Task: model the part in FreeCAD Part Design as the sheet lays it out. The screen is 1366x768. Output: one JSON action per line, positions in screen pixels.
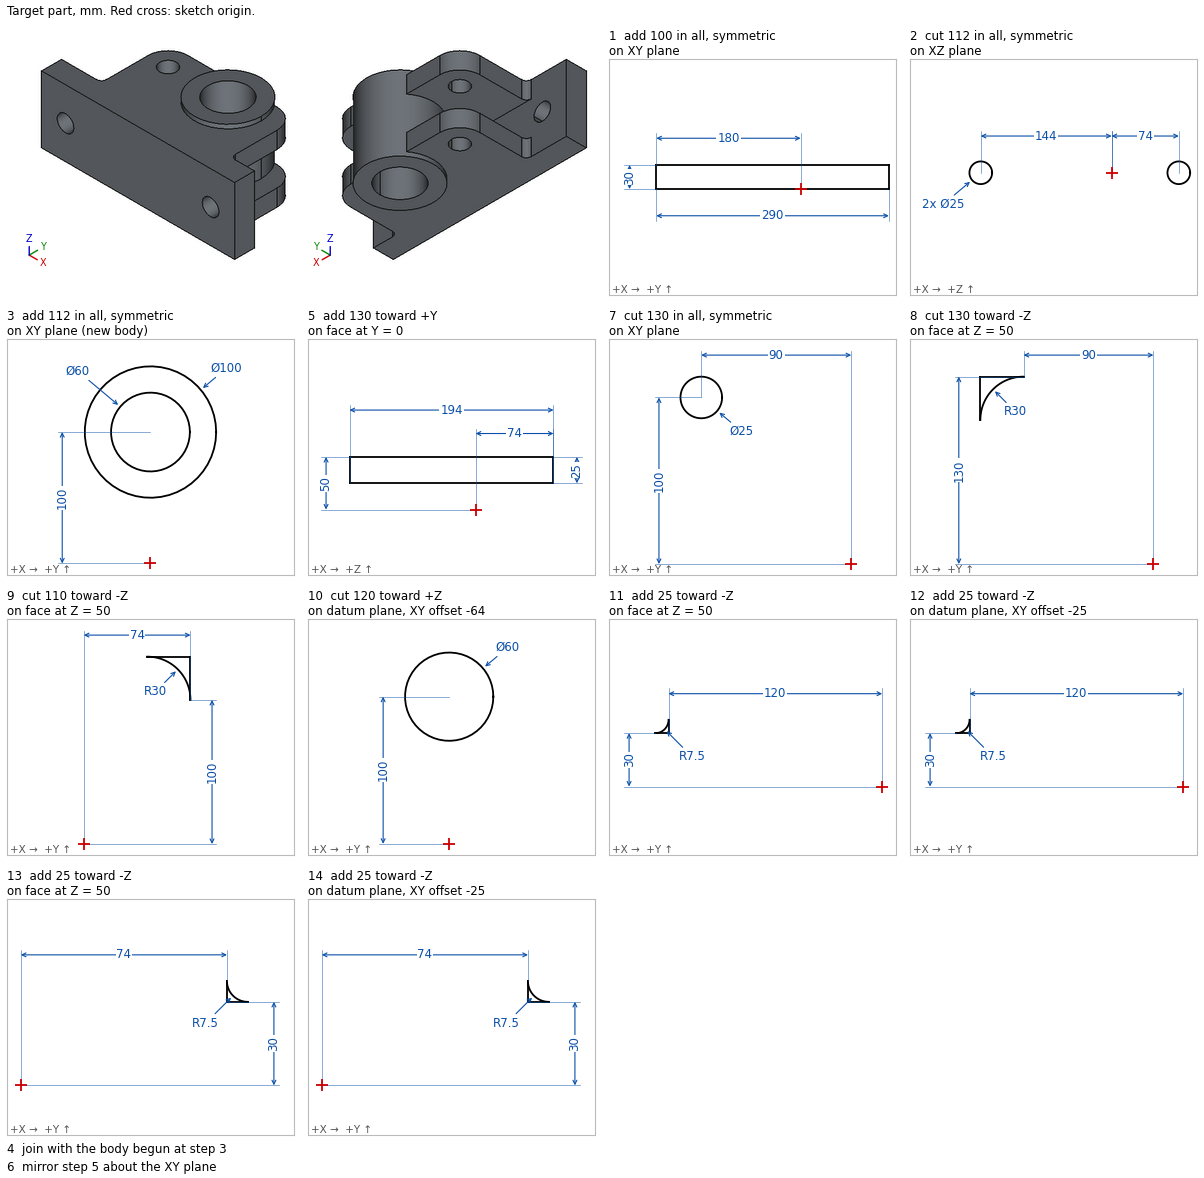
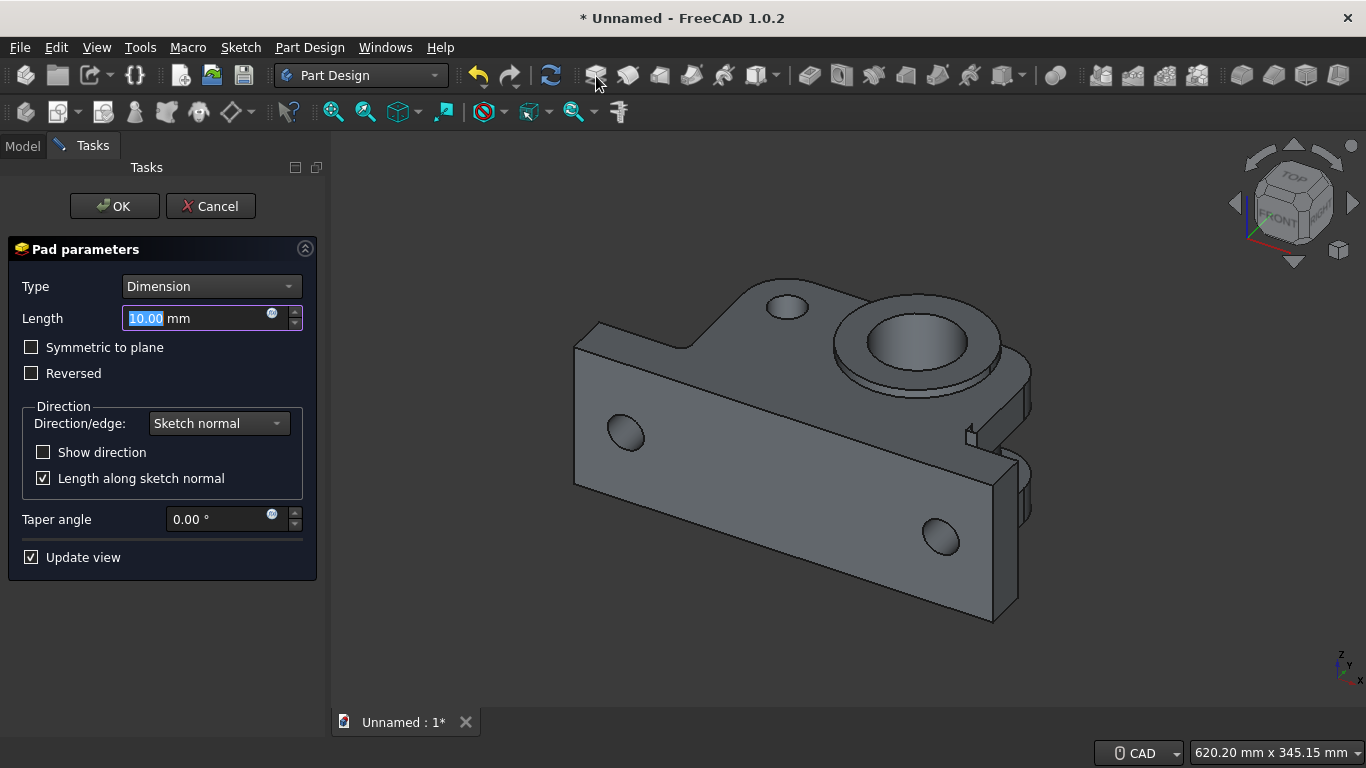
{"action": "type", "text": "25"}
{"action": "key", "text": "Tab"}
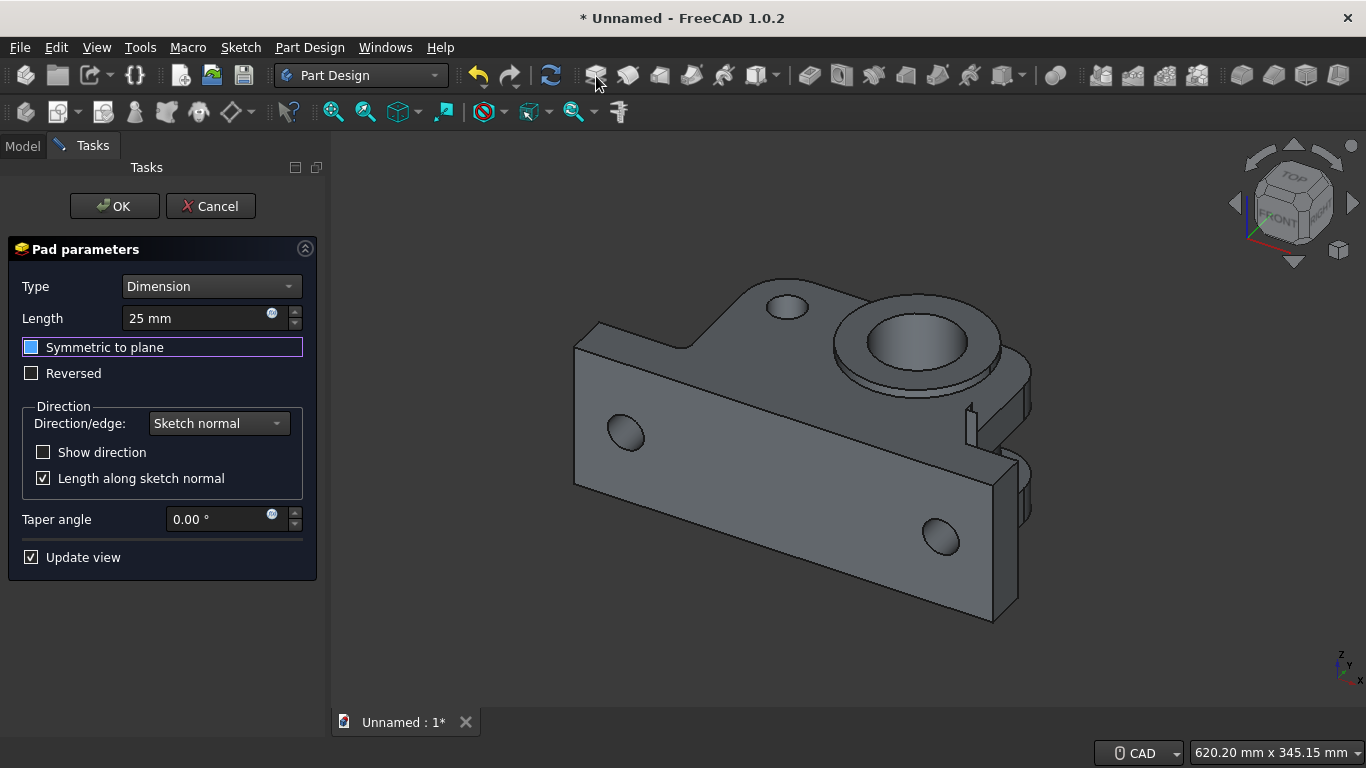
{"action": "left_click", "coordinate": [30, 373]}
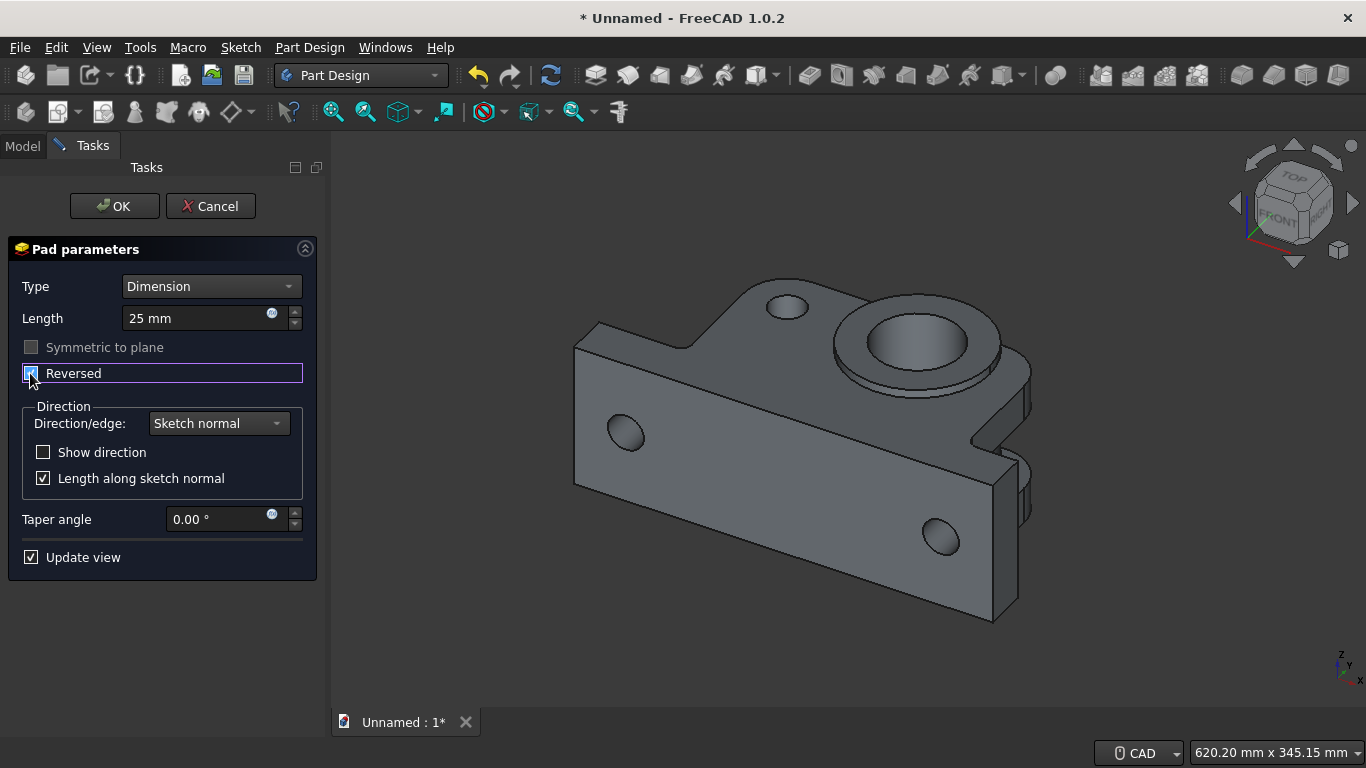
{"action": "left_click", "coordinate": [115, 206]}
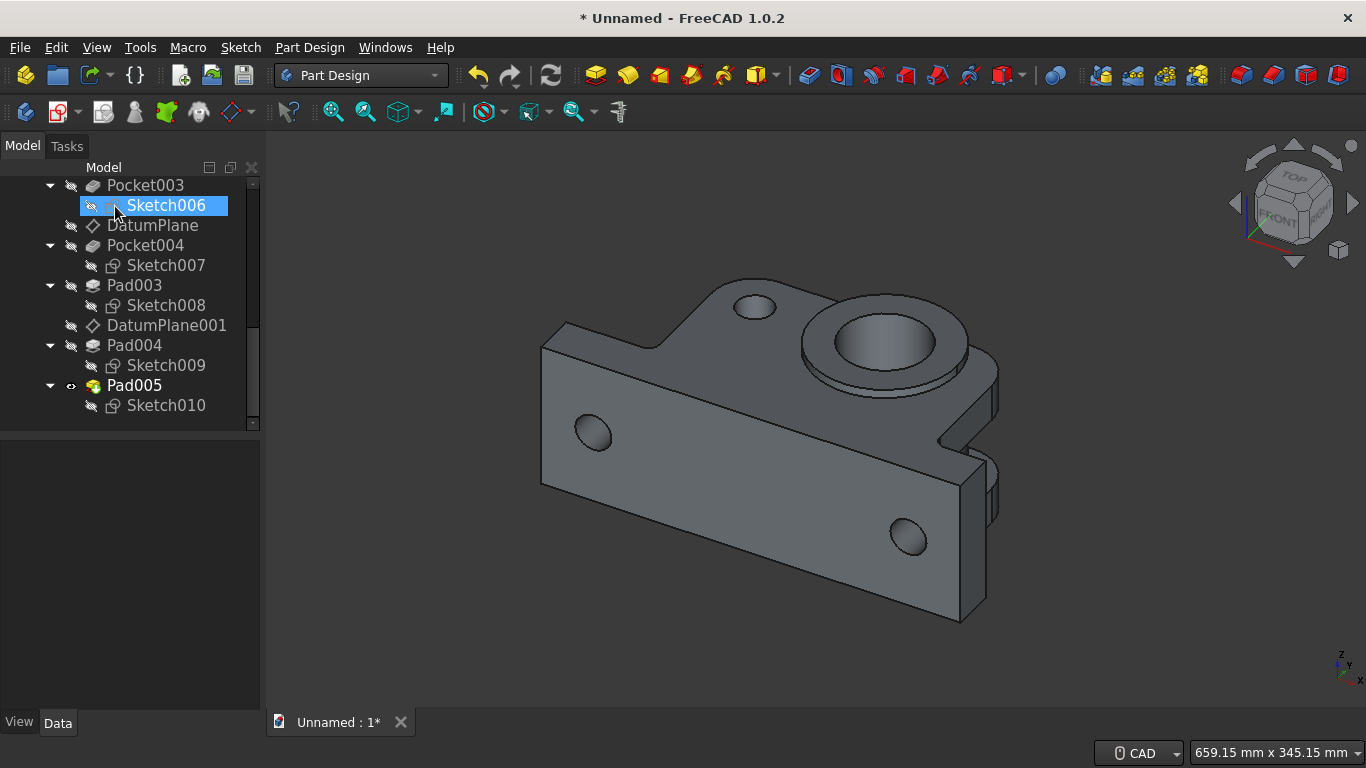
{"action": "scroll", "coordinate": [140, 301], "scroll_direction": "down", "scroll_amount": 3}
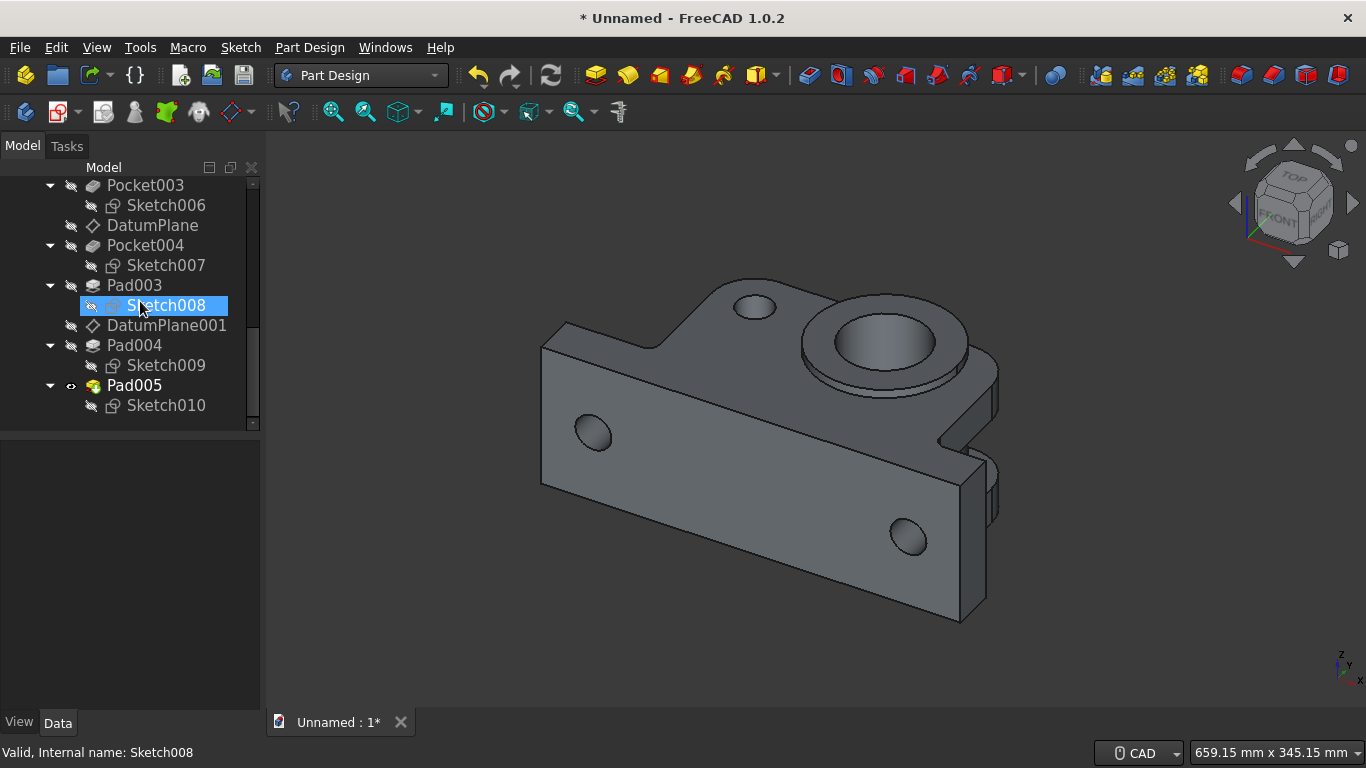
{"action": "scroll", "coordinate": [140, 301], "scroll_direction": "up", "scroll_amount": 15}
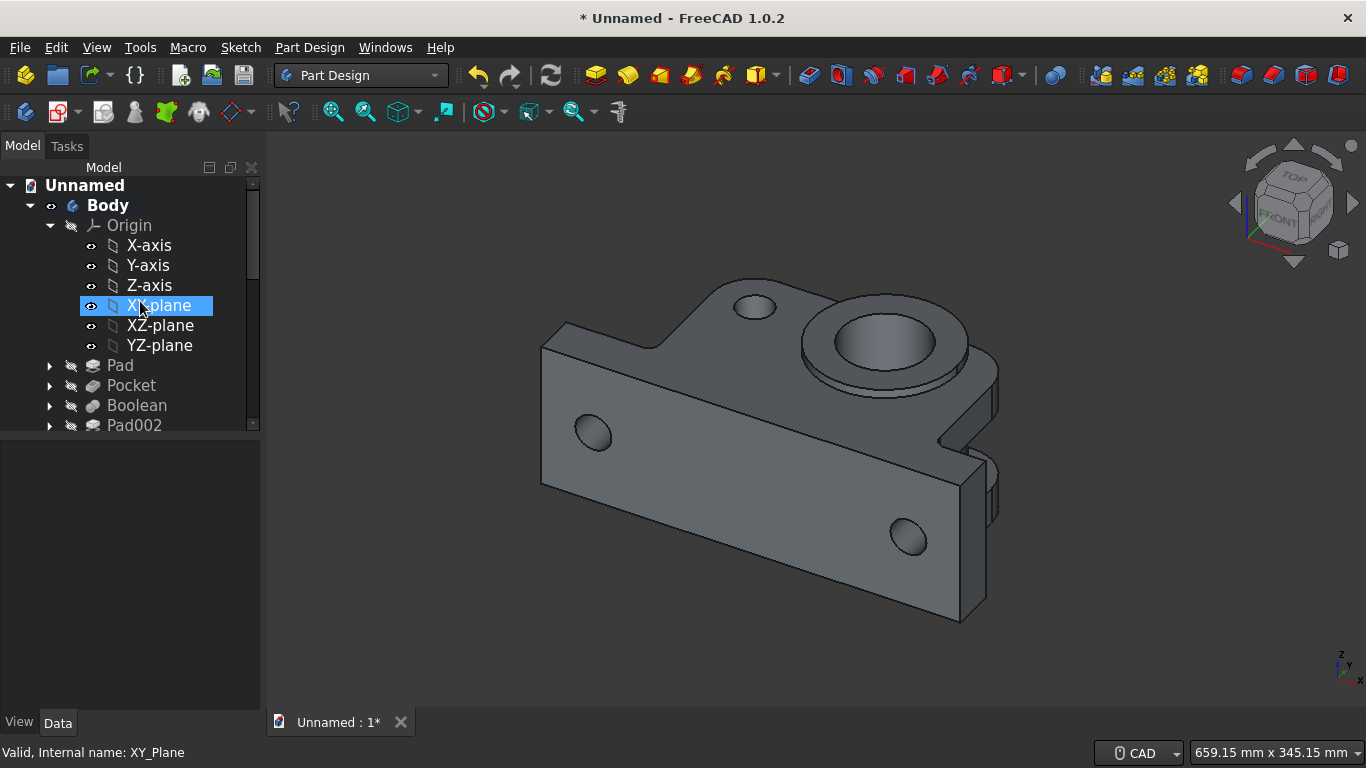
{"action": "left_click", "coordinate": [136, 306]}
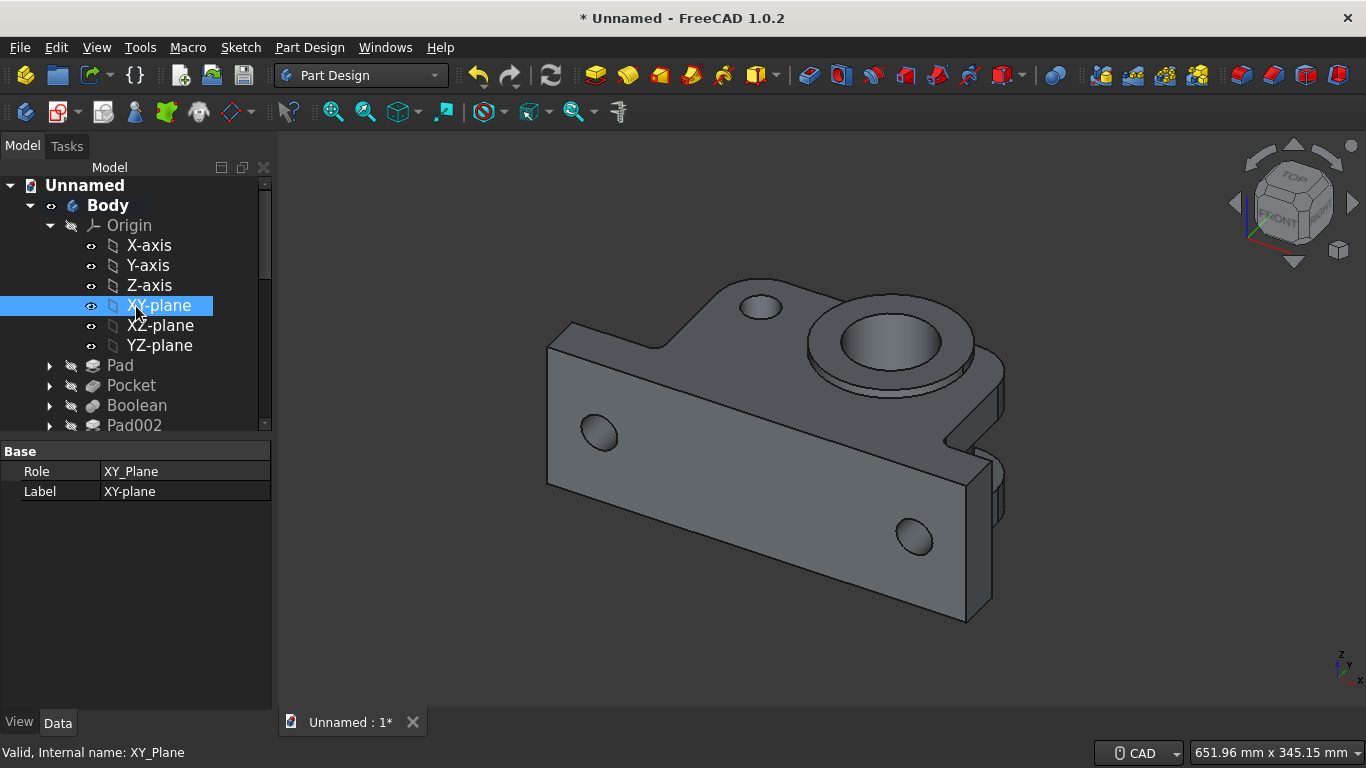
{"action": "left_click", "coordinate": [232, 112]}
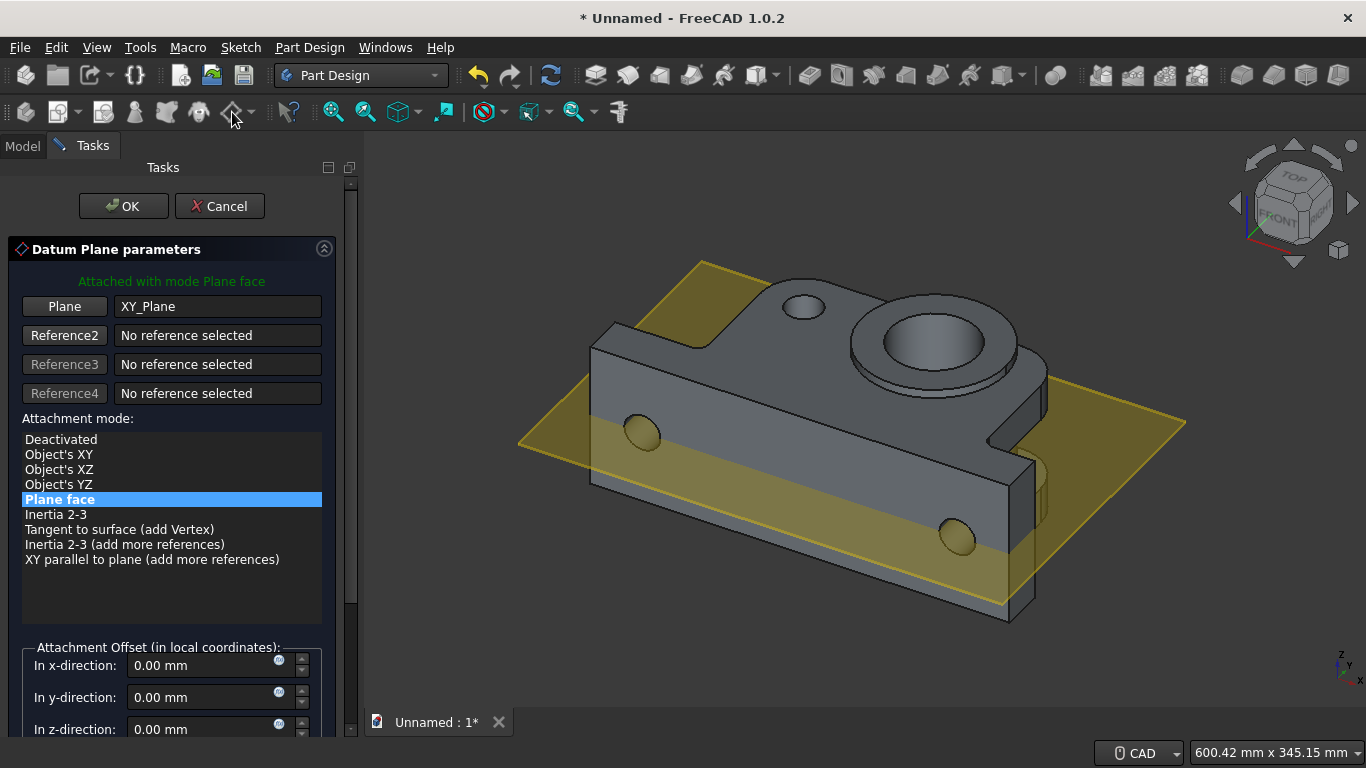
{"action": "scroll", "coordinate": [351, 456], "scroll_direction": "down", "scroll_amount": 2}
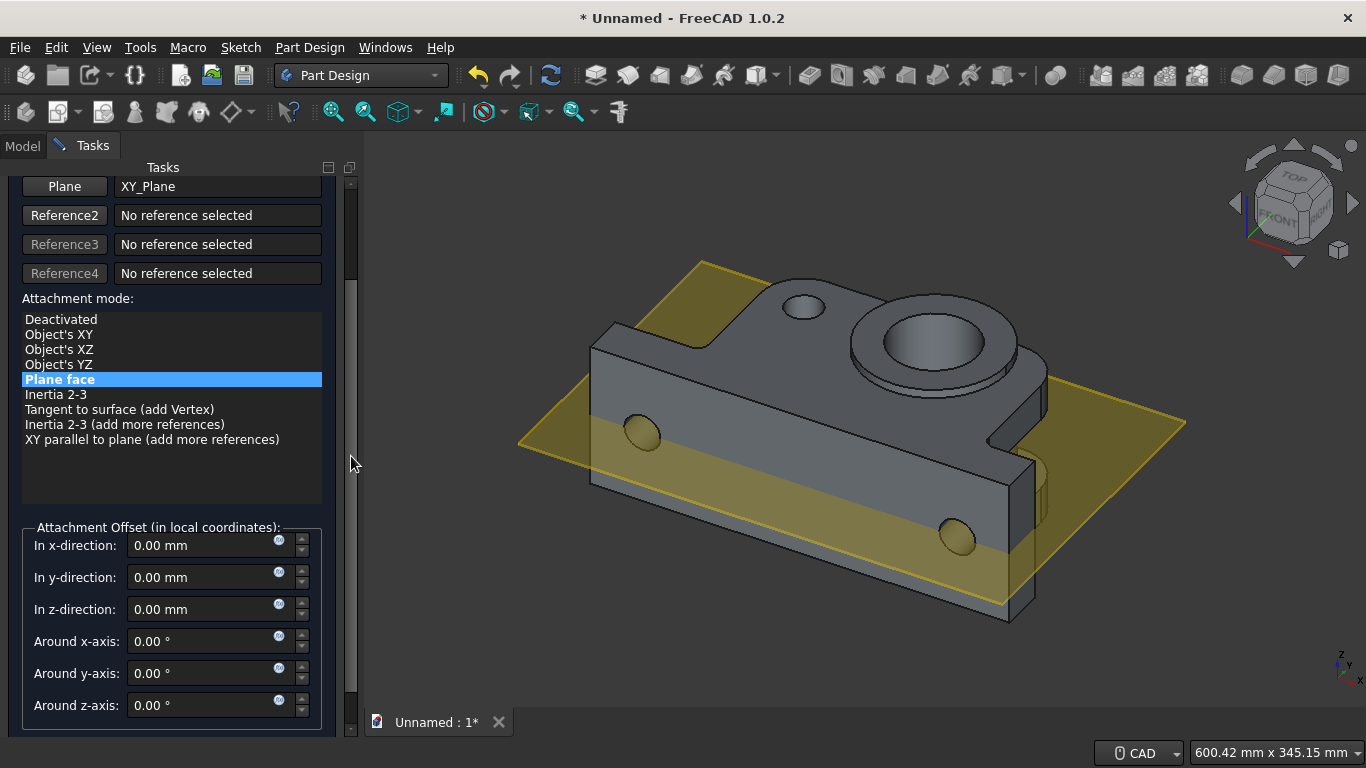
{"action": "triple_click", "coordinate": [210, 609]}